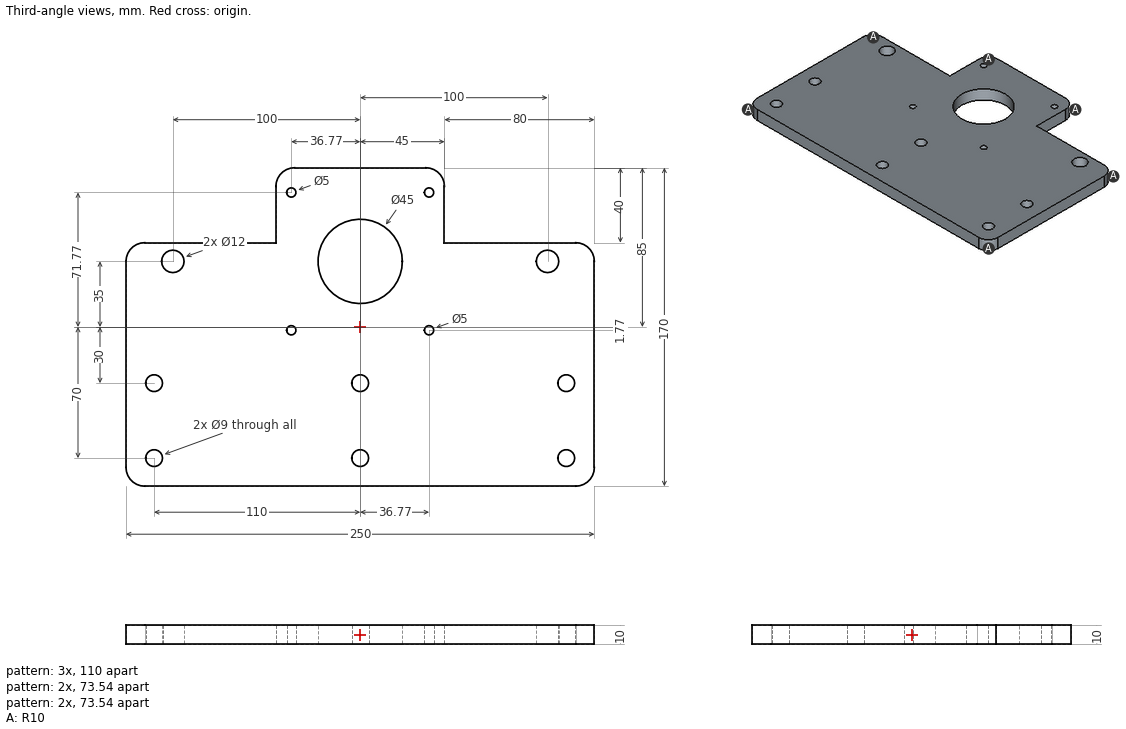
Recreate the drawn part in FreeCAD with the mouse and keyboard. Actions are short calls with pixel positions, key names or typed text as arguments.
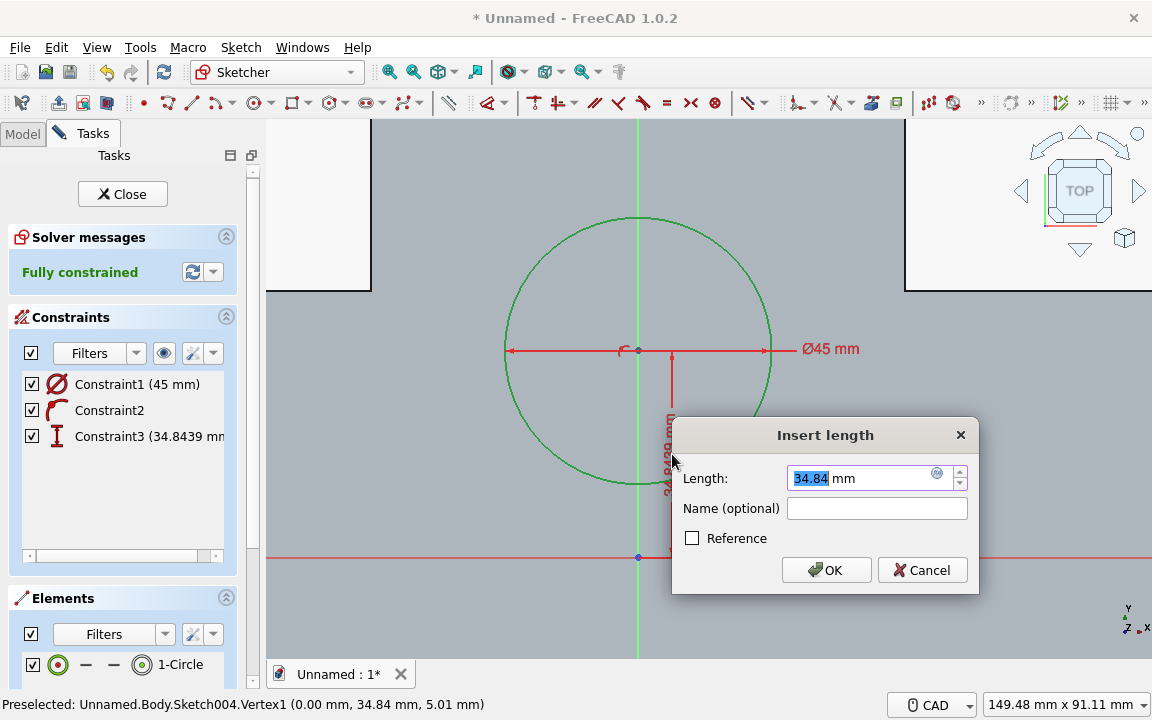
text(35)
key(Return)
key(Escape)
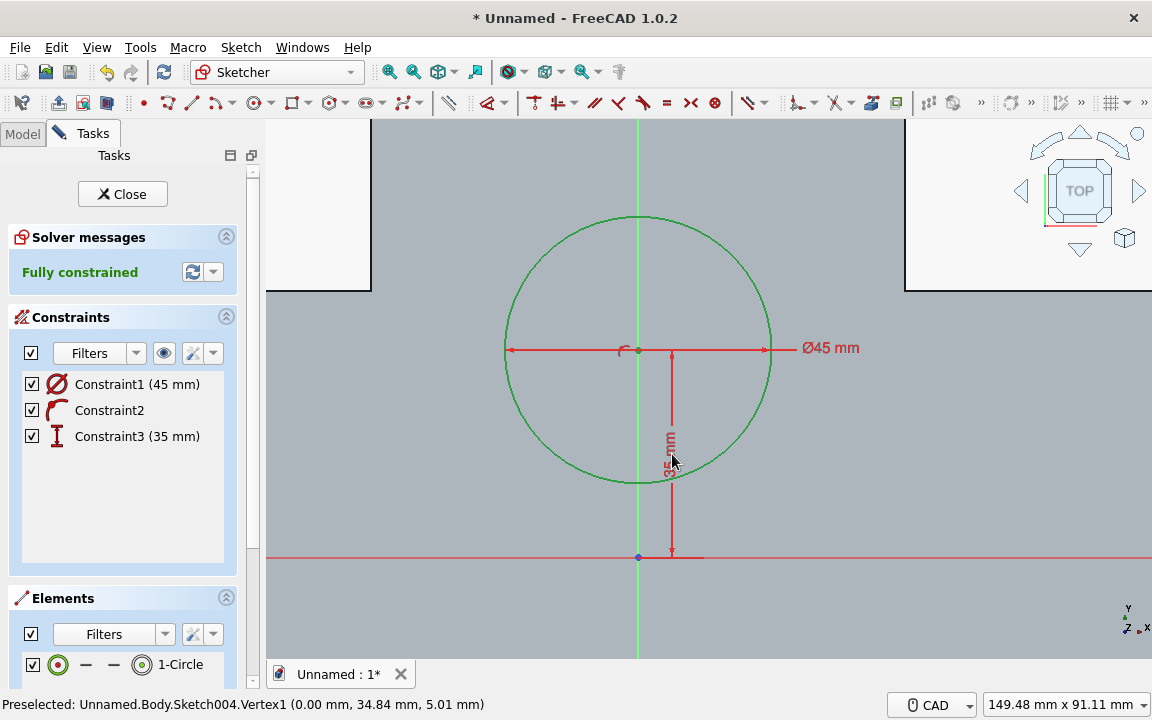
click(123, 194)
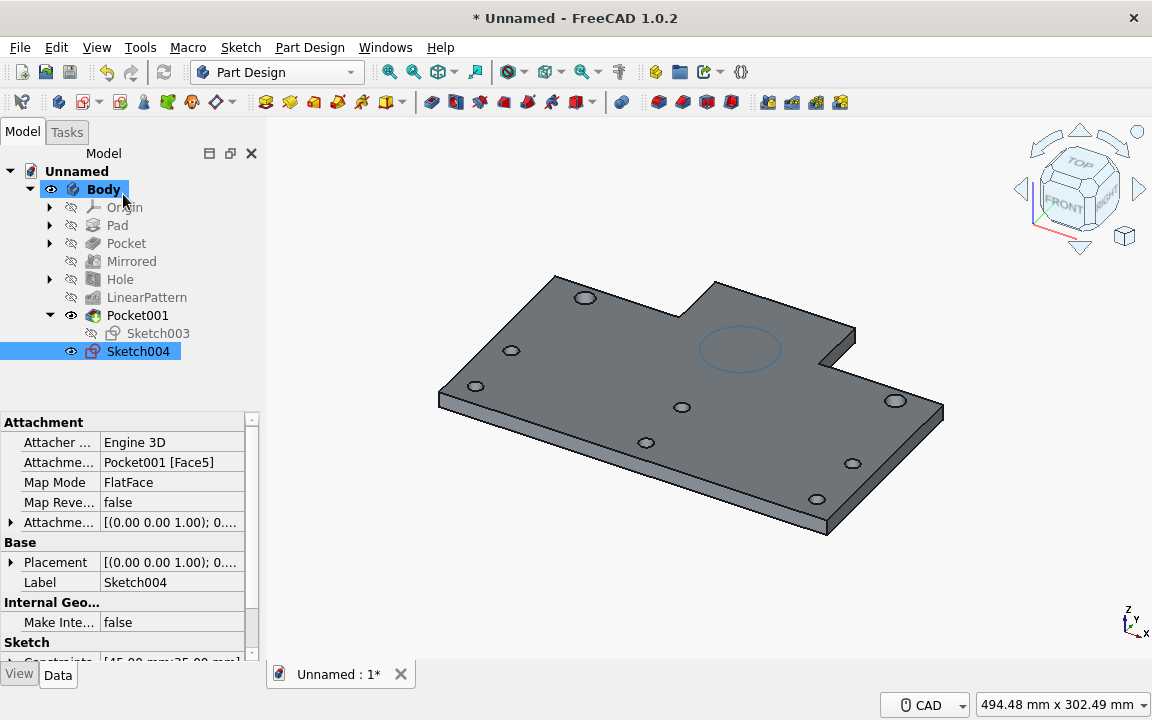
click(432, 102)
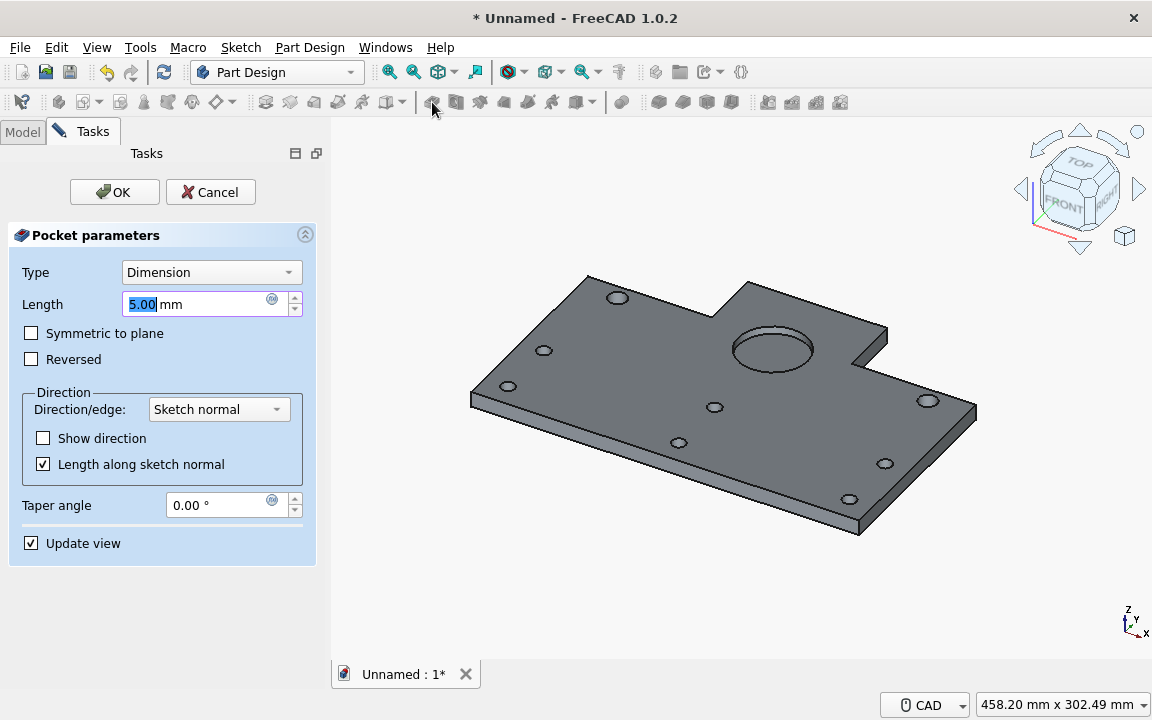
text(10)
key(Tab)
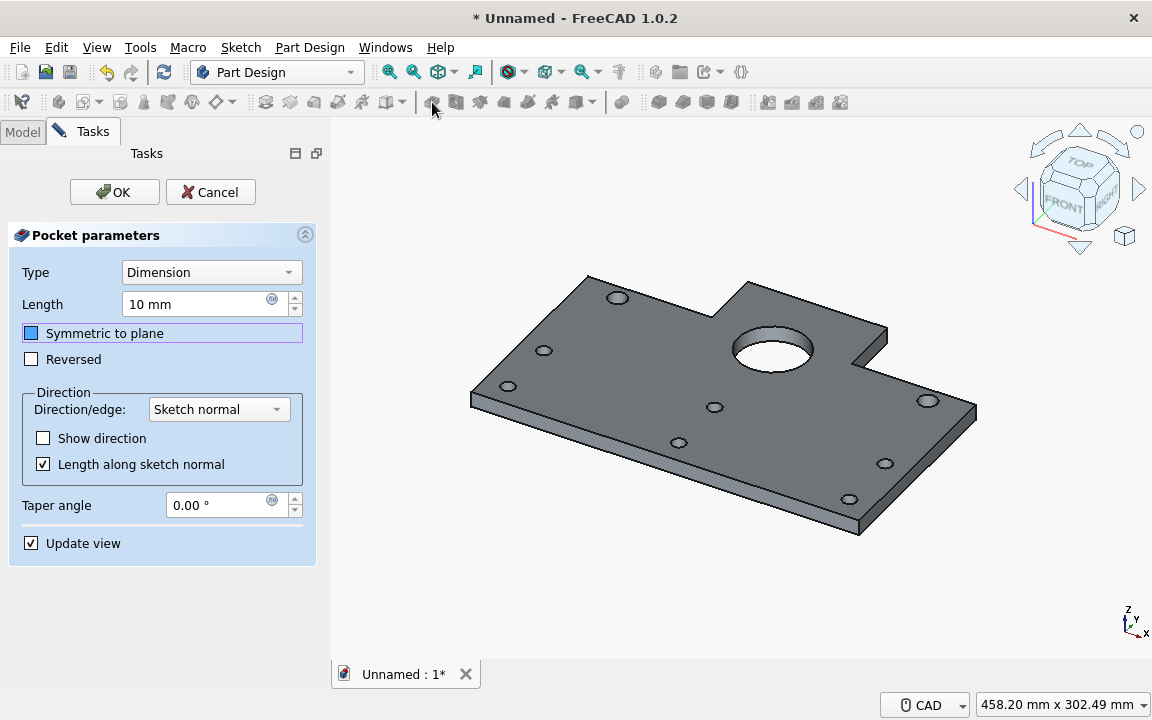
click(115, 192)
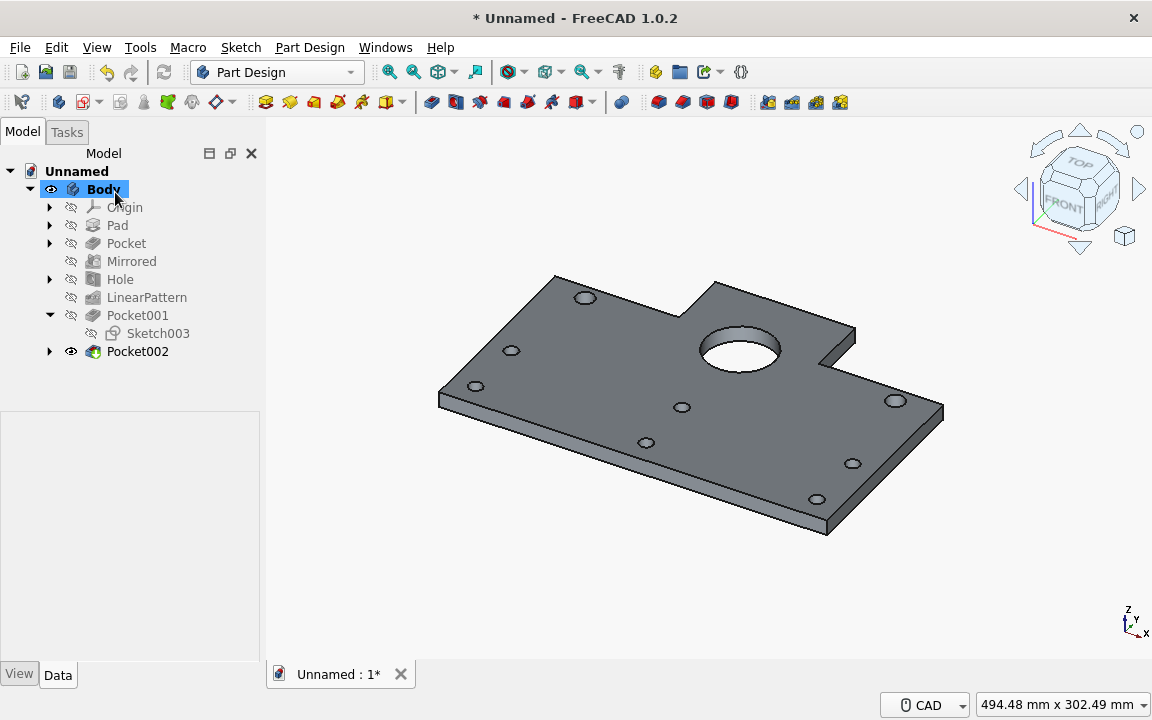
click(820, 416)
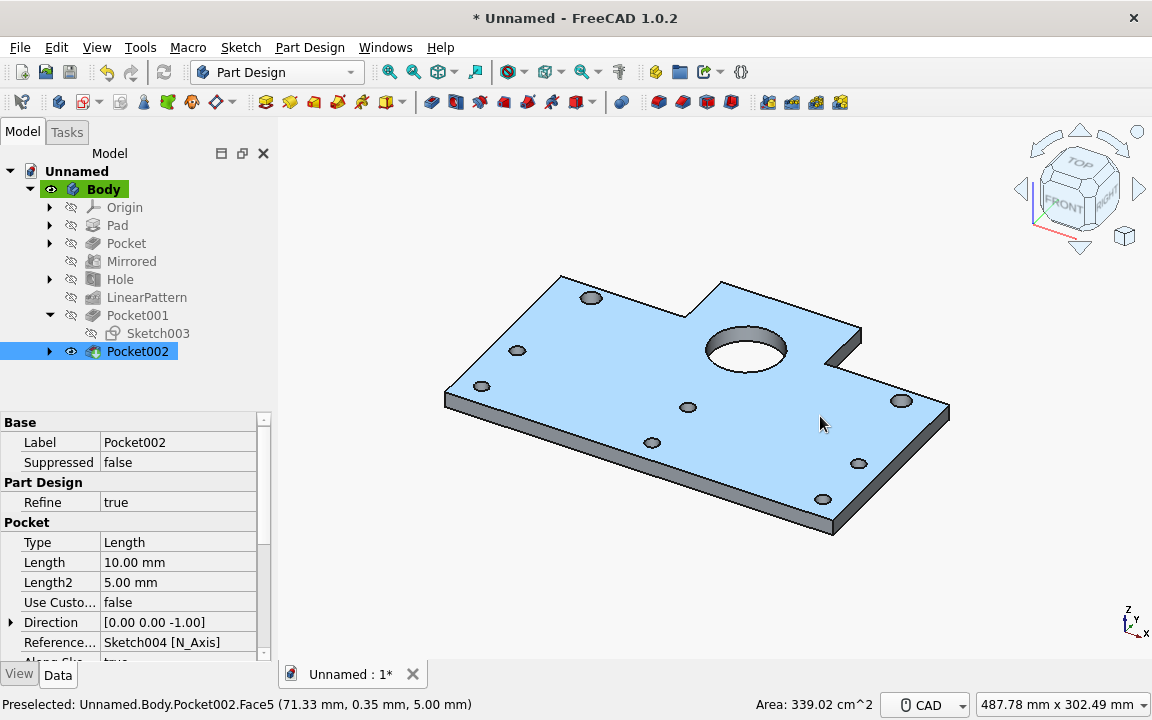
click(84, 102)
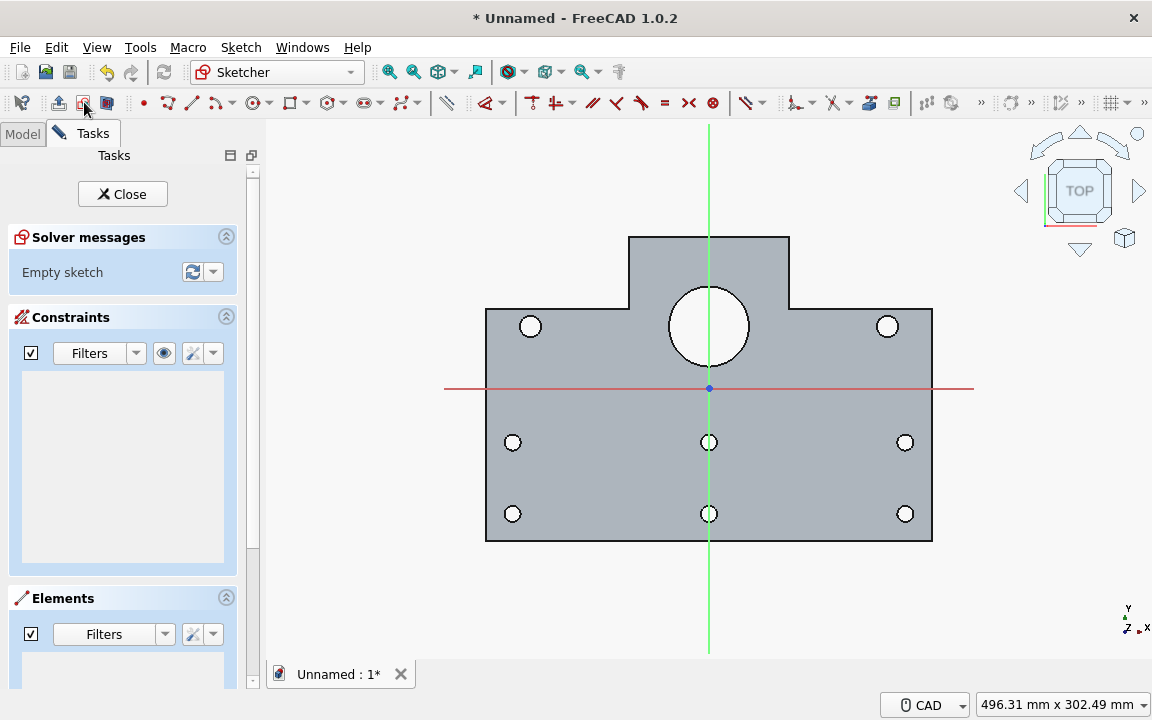
scroll(644, 254, up, 15)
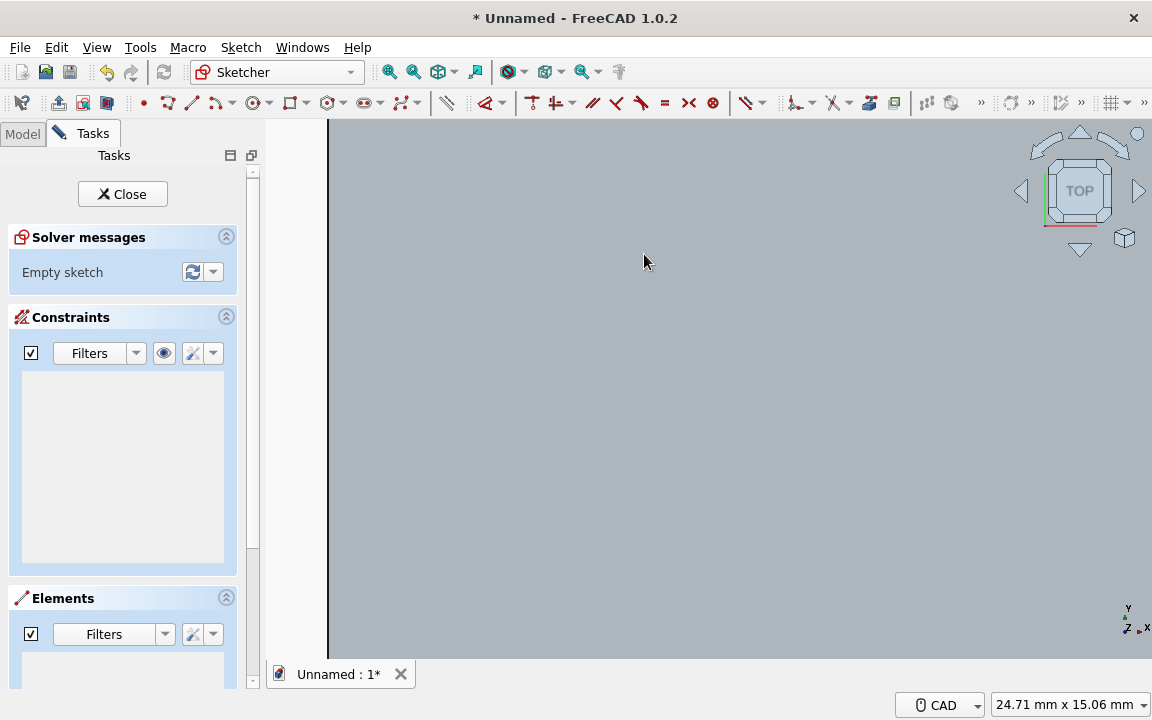
scroll(602, 385, up, 3)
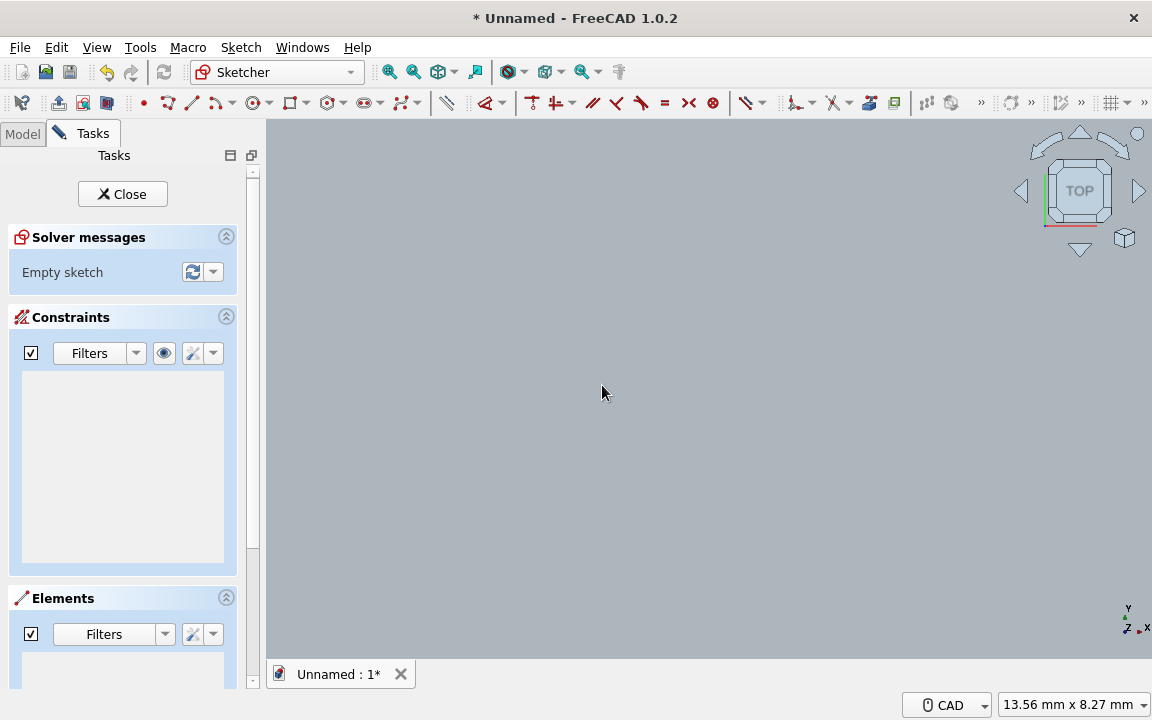
key(g)
key(c)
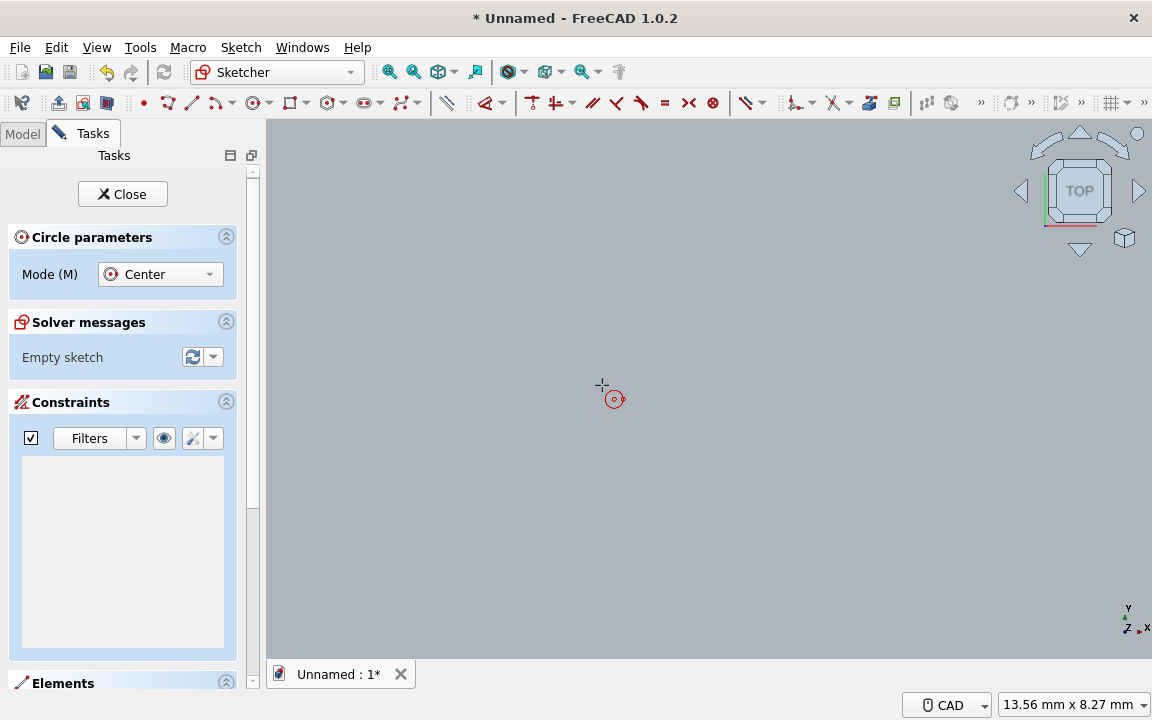
click(640, 389)
move(755, 273)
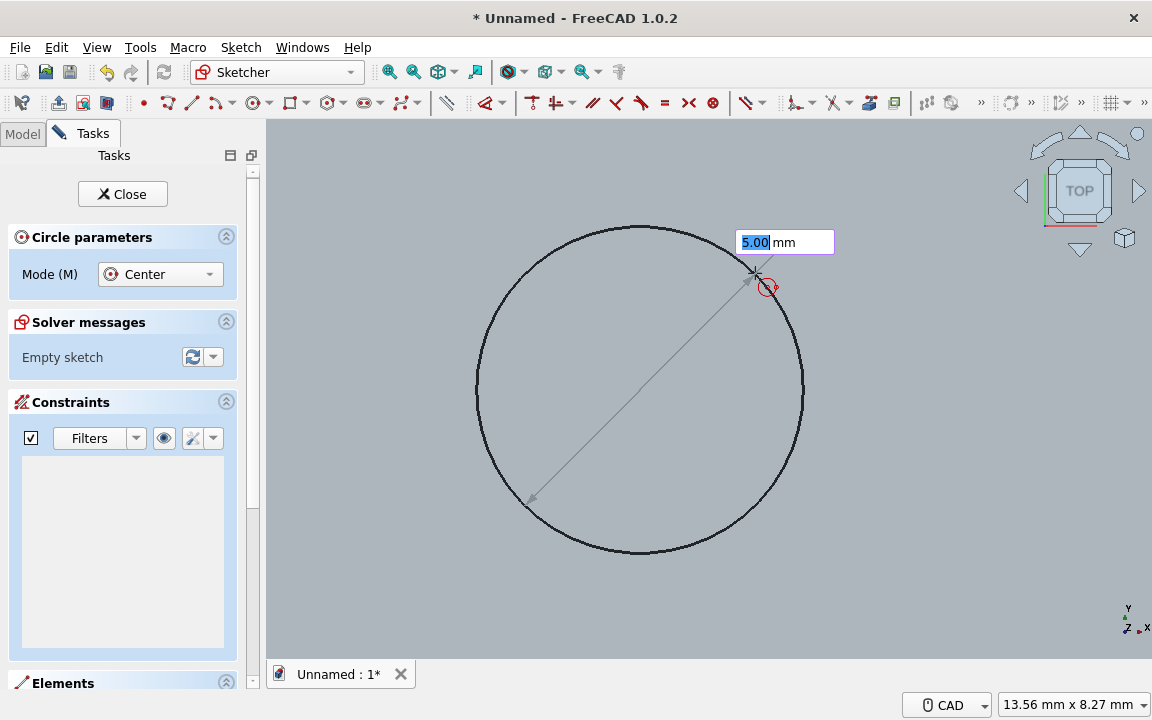
text(5)
key(Return)
key(Escape)